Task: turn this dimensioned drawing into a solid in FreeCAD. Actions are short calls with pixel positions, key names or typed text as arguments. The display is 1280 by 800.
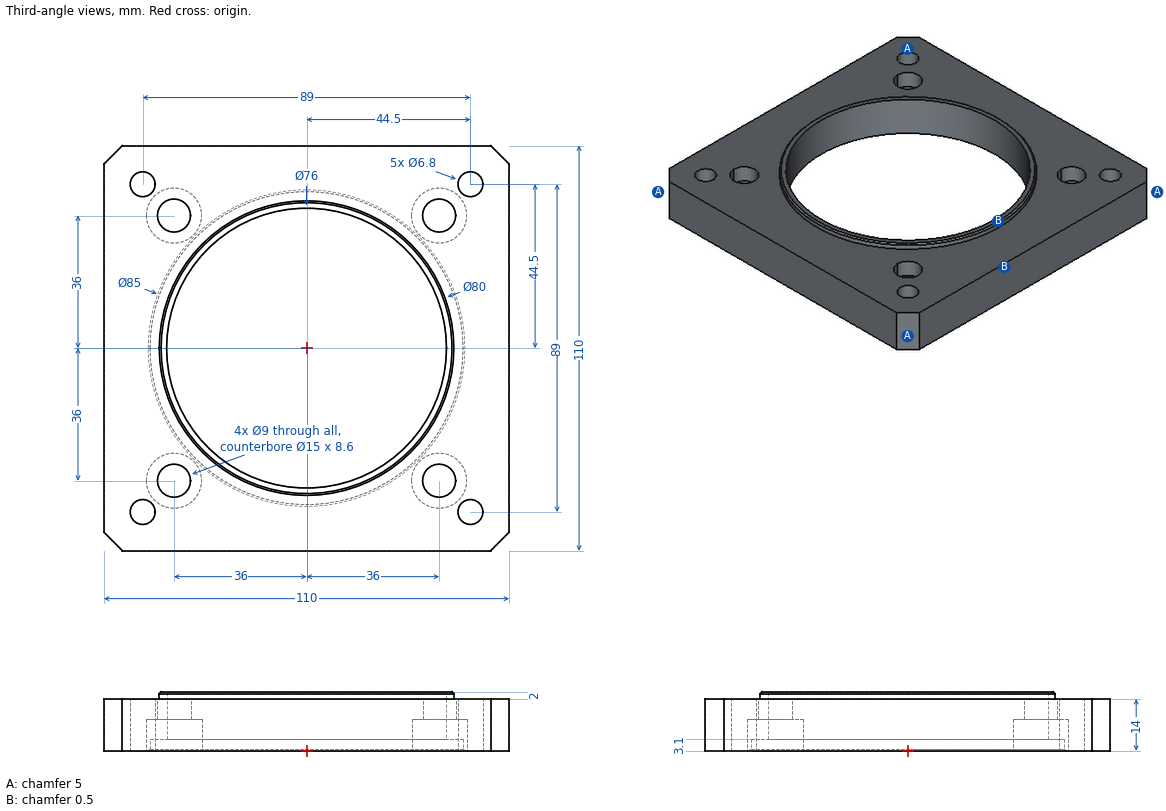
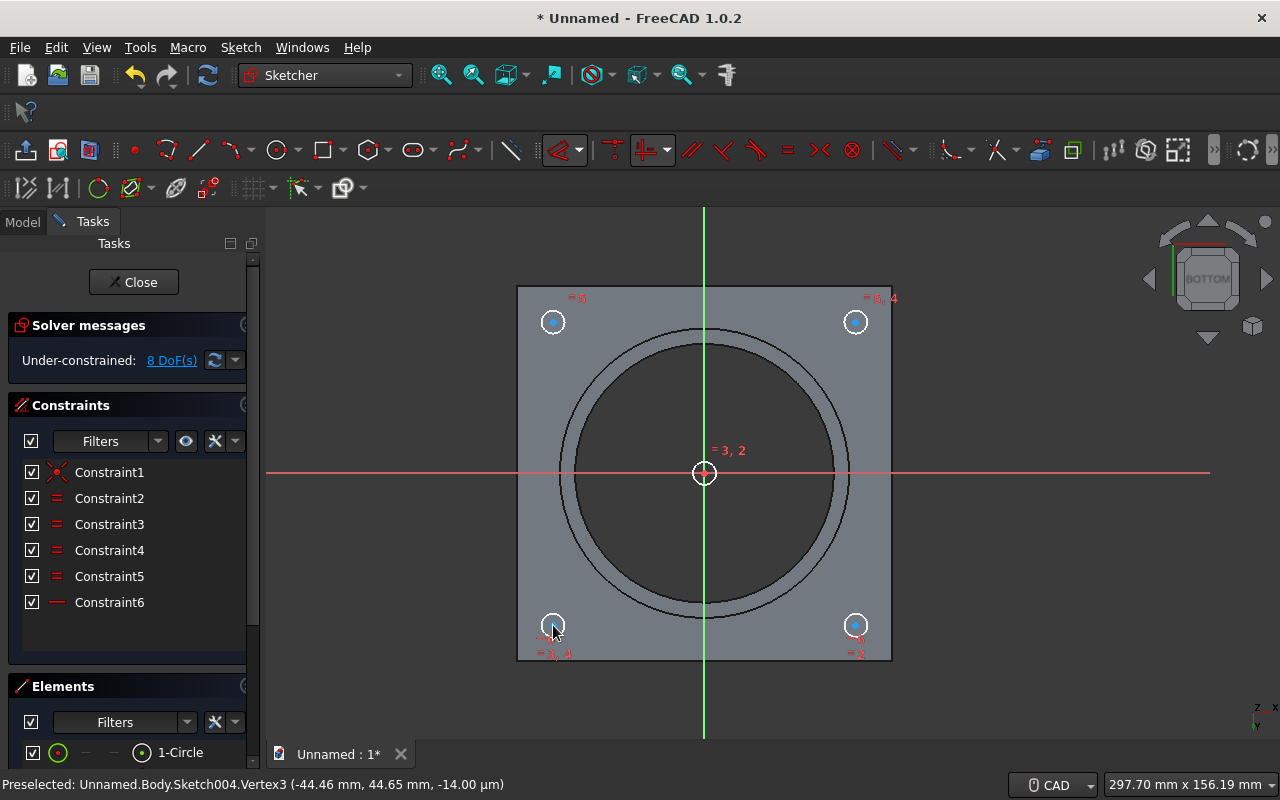
click(856, 625)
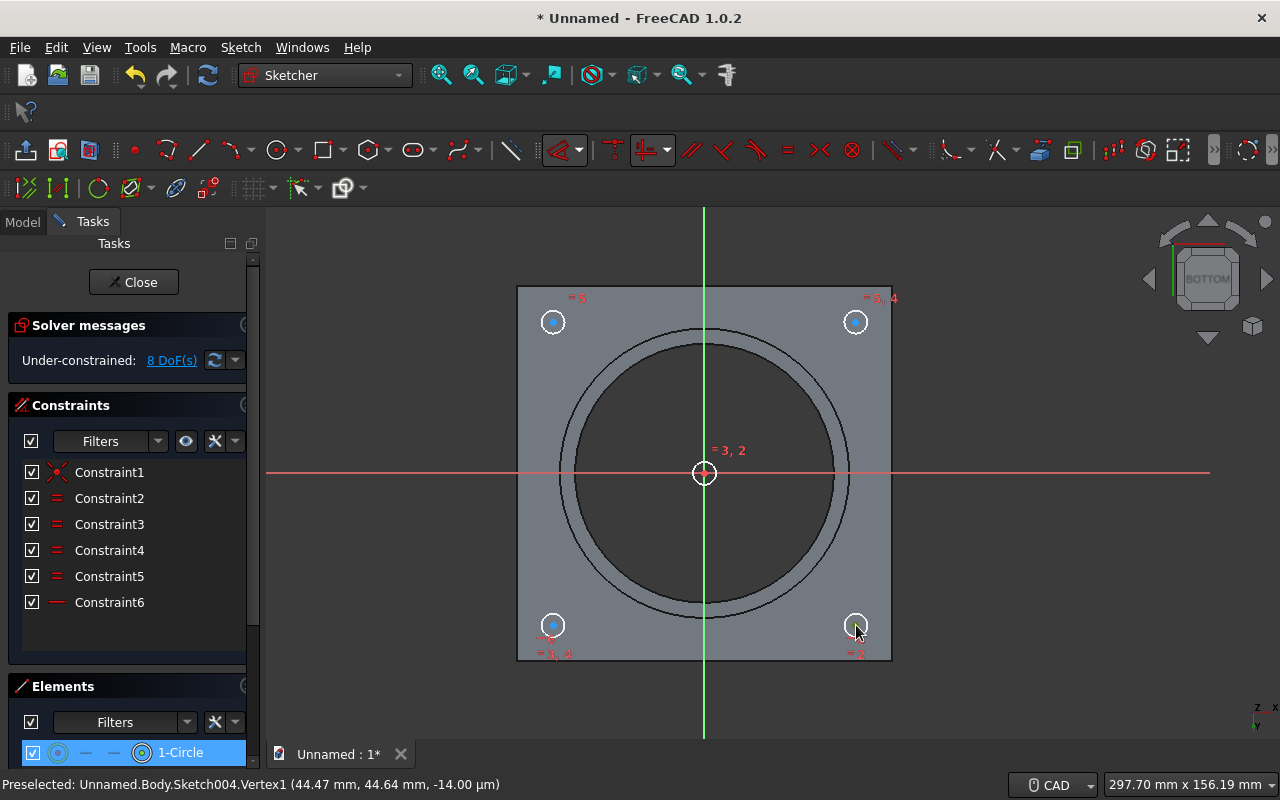
click(856, 322)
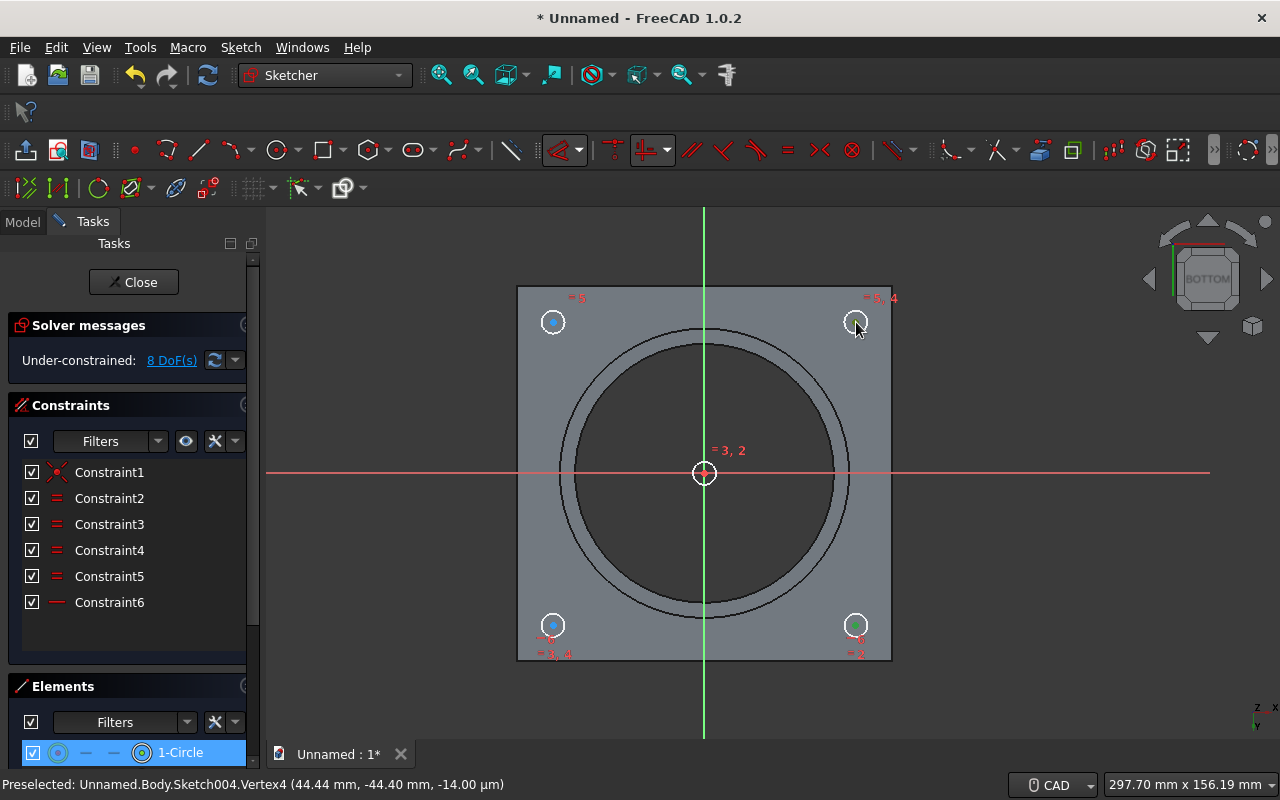
click(670, 150)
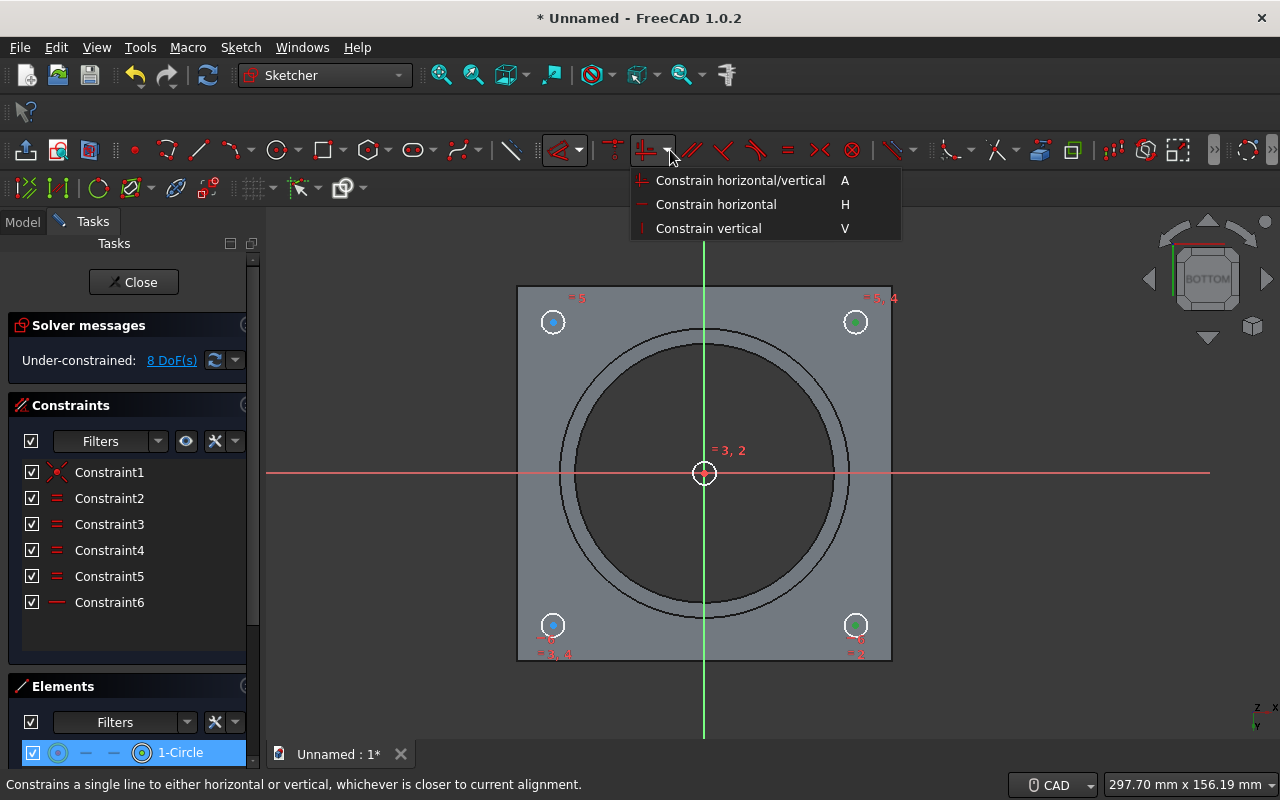
click(766, 228)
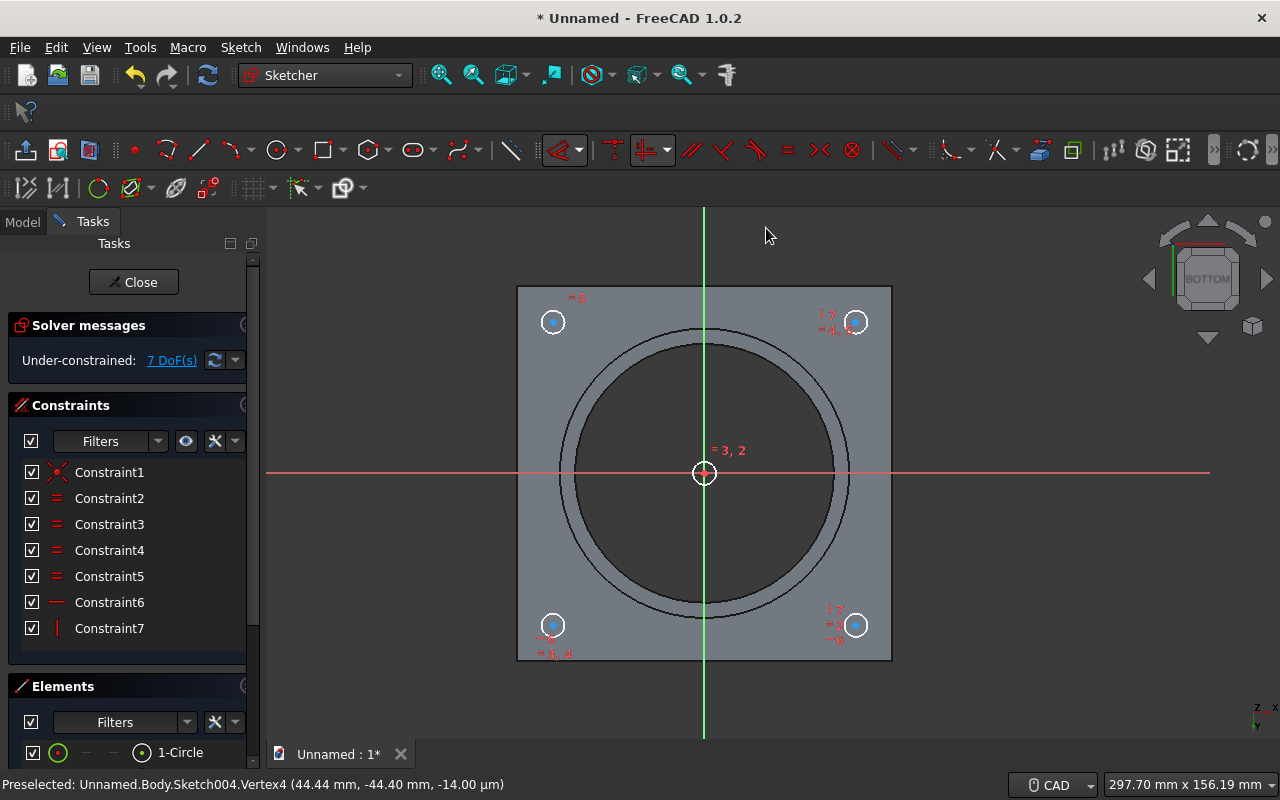
click(553, 625)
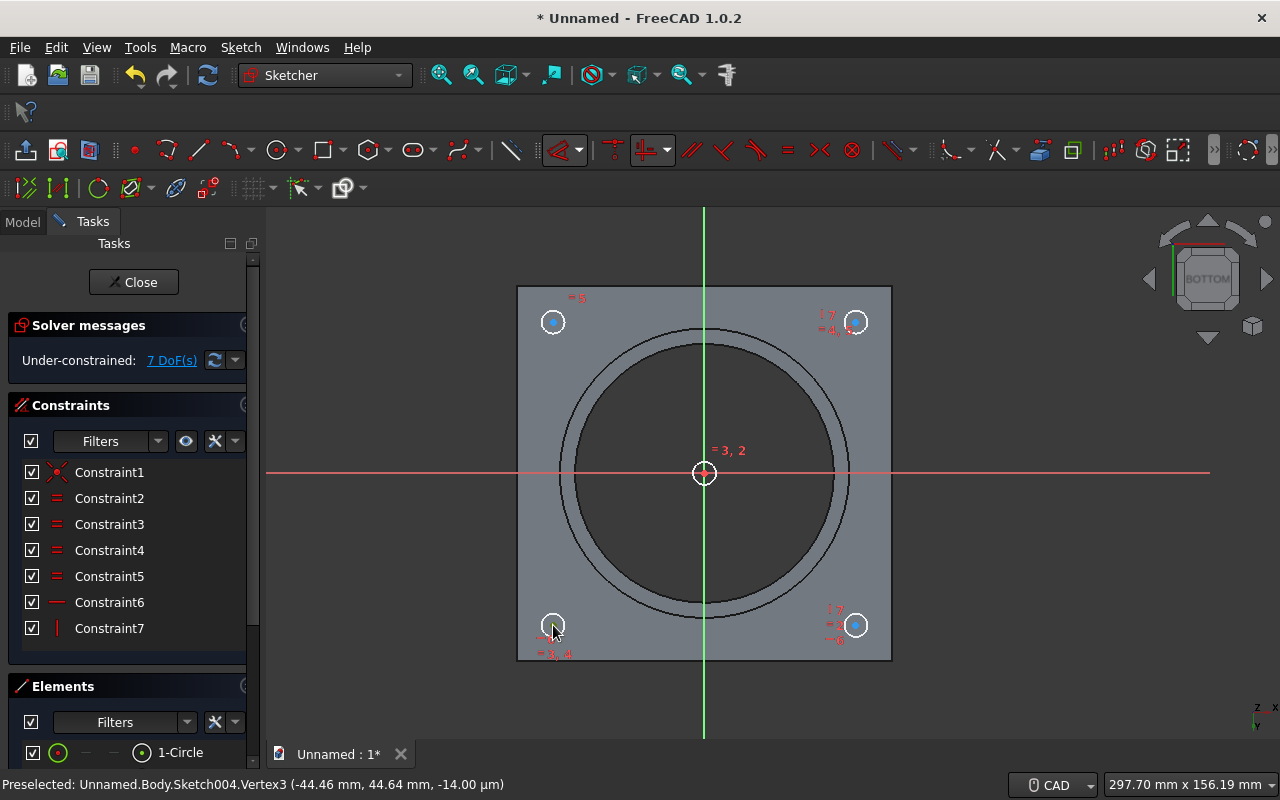
click(553, 322)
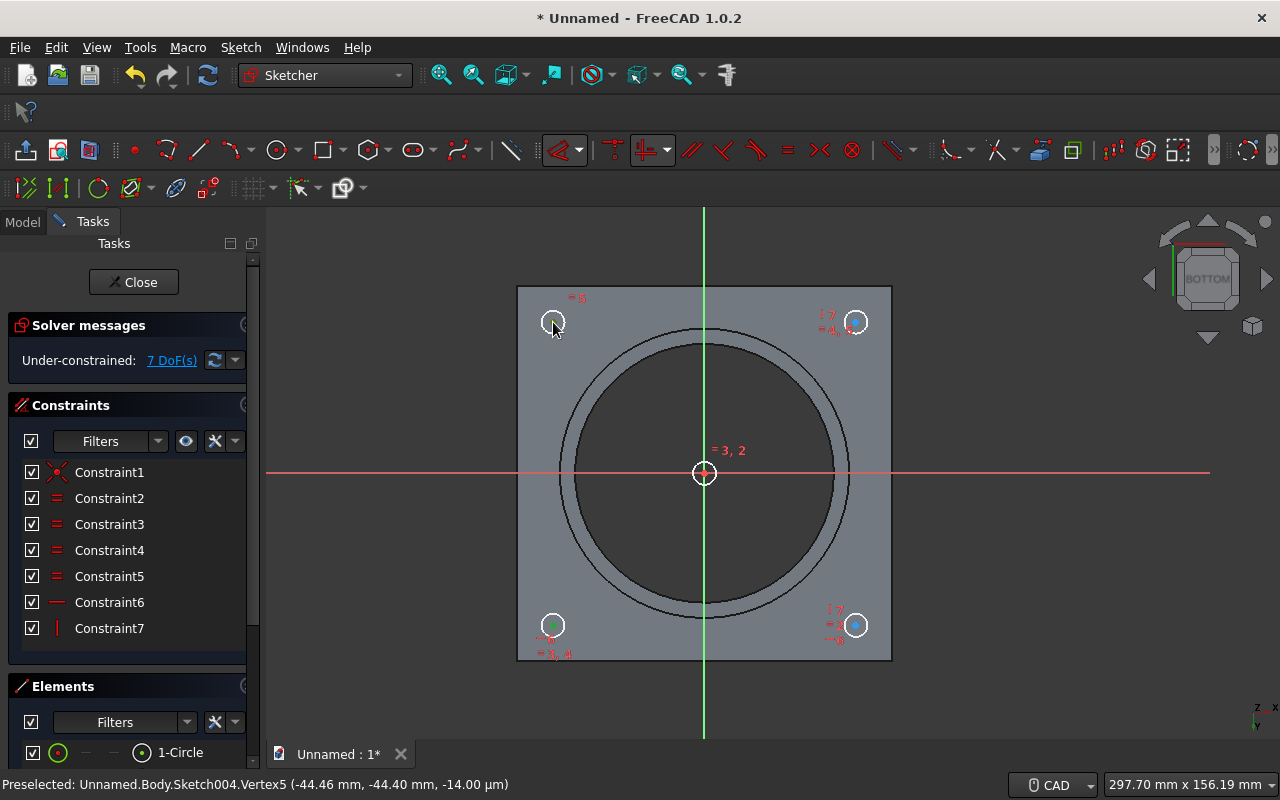
click(670, 150)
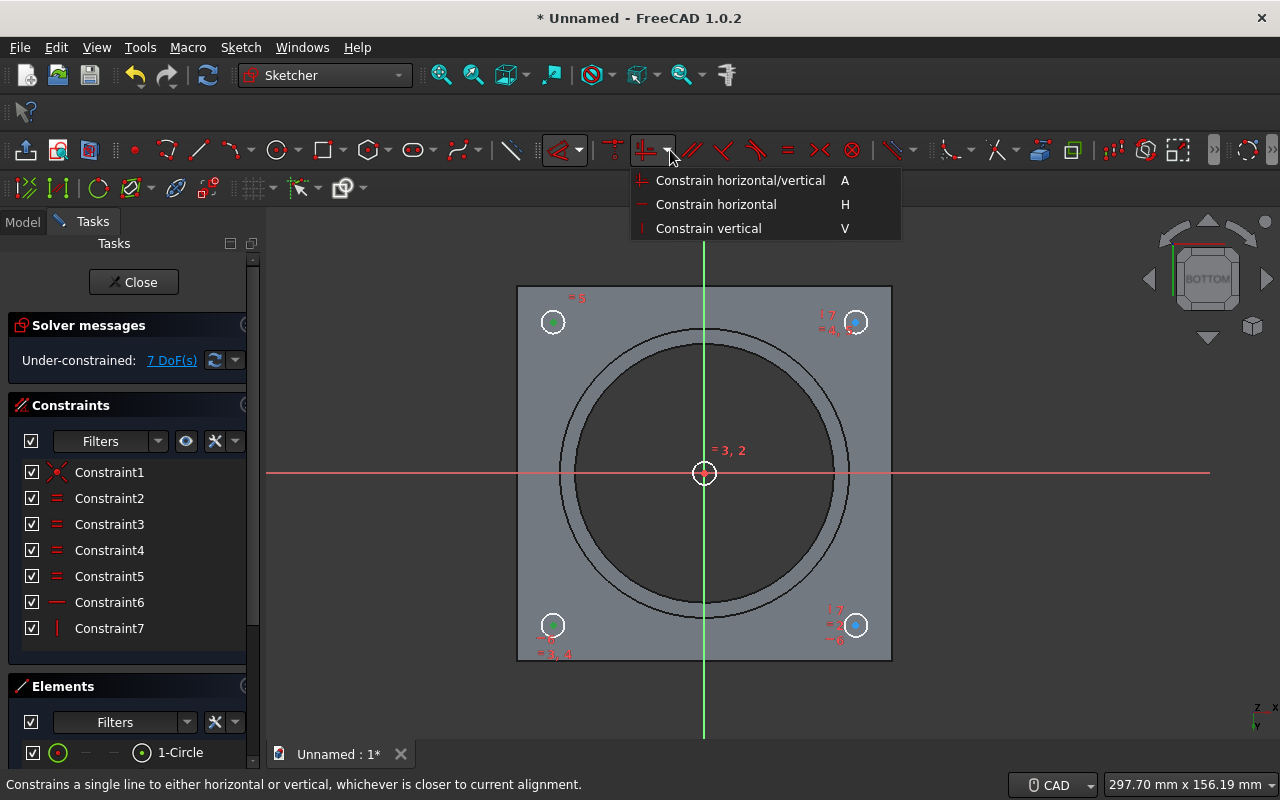
click(766, 228)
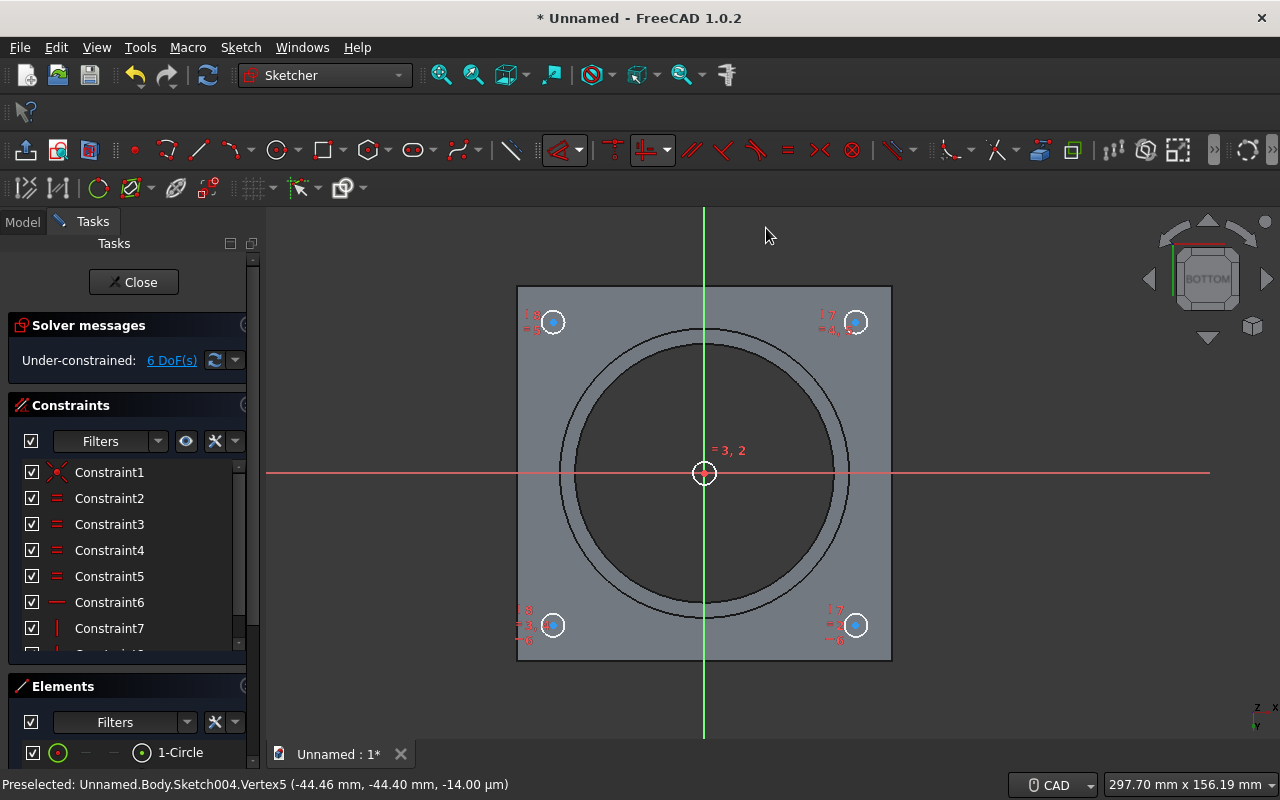
click(856, 322)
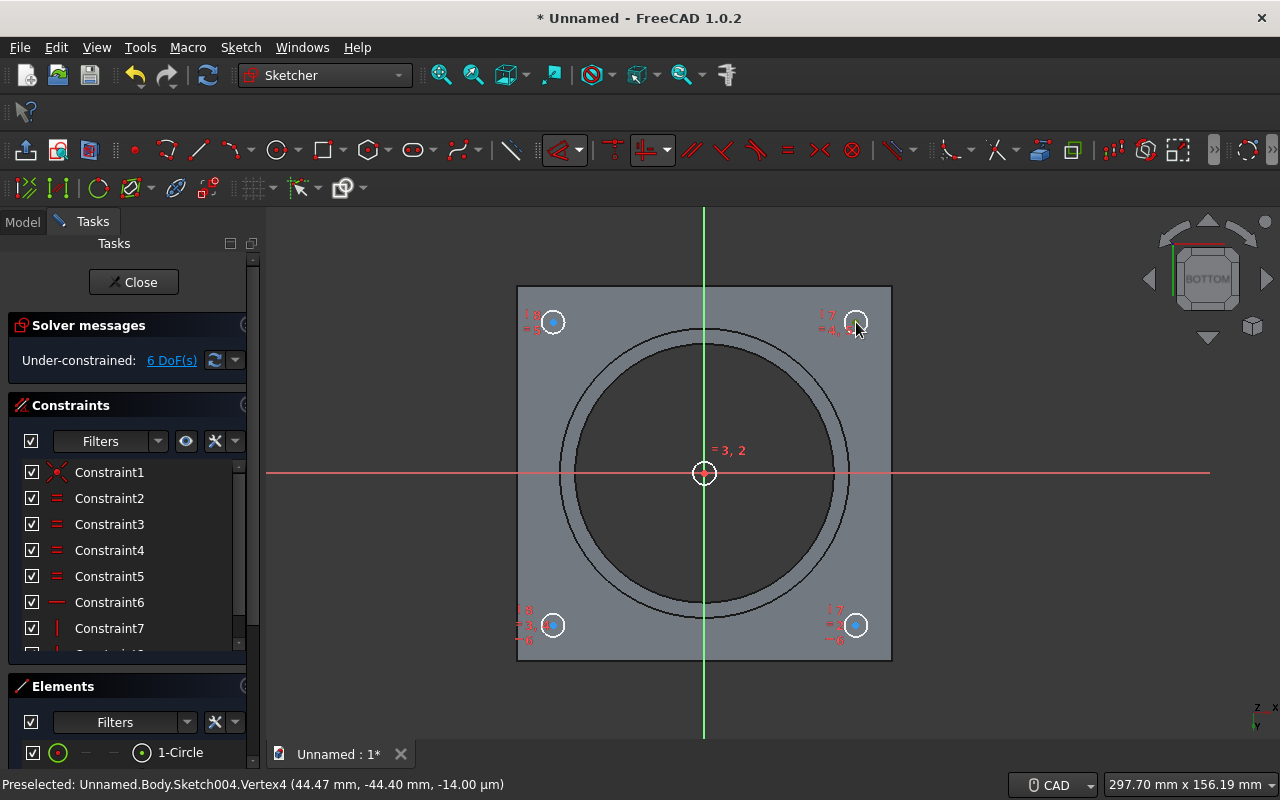
click(553, 322)